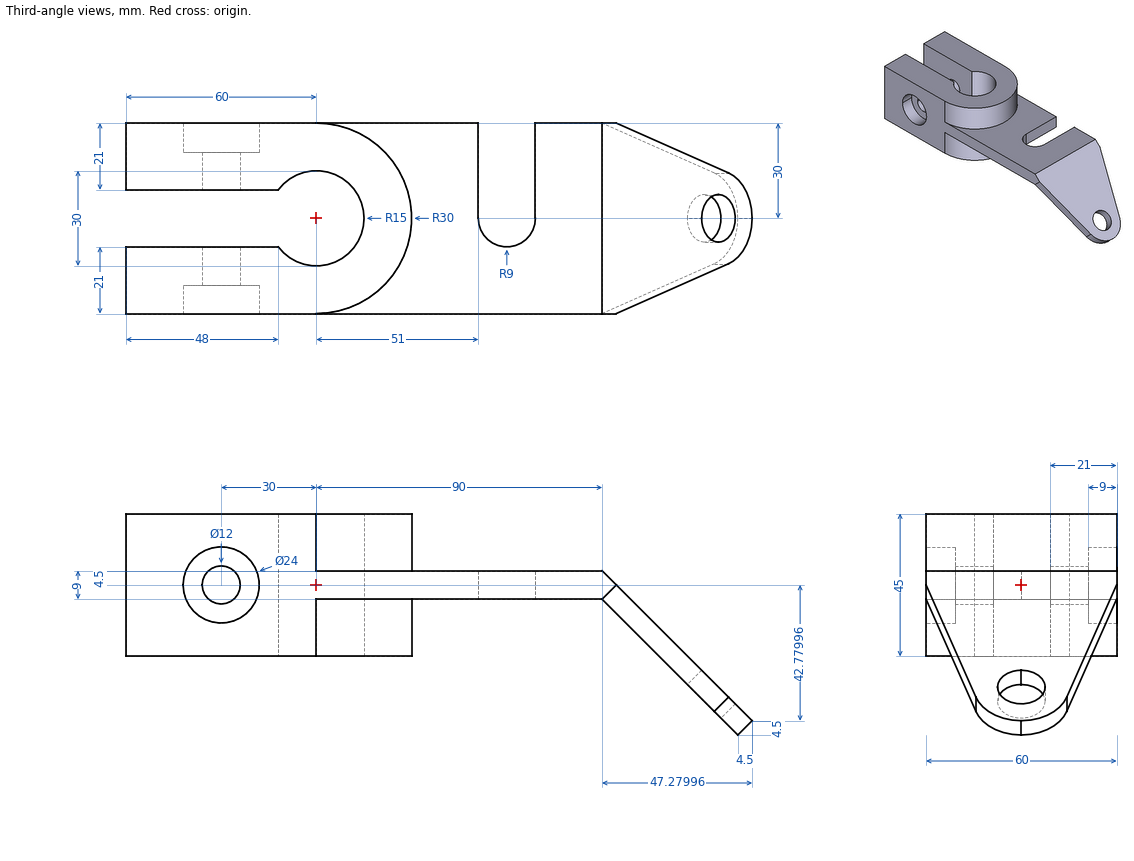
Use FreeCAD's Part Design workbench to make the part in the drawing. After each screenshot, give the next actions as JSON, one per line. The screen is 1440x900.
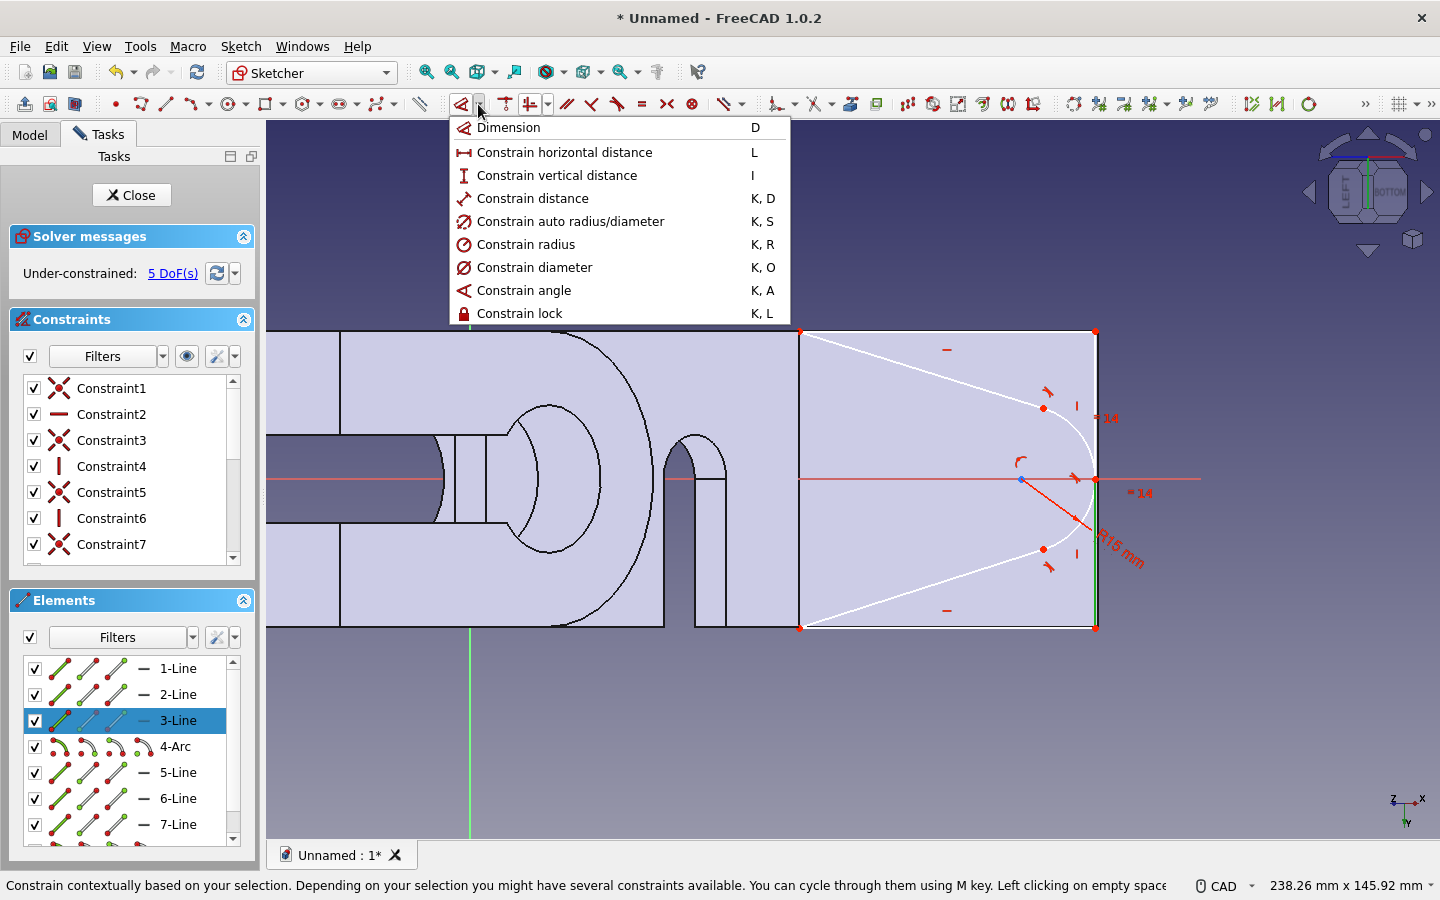
{"action": "left_click", "coordinate": [620, 176]}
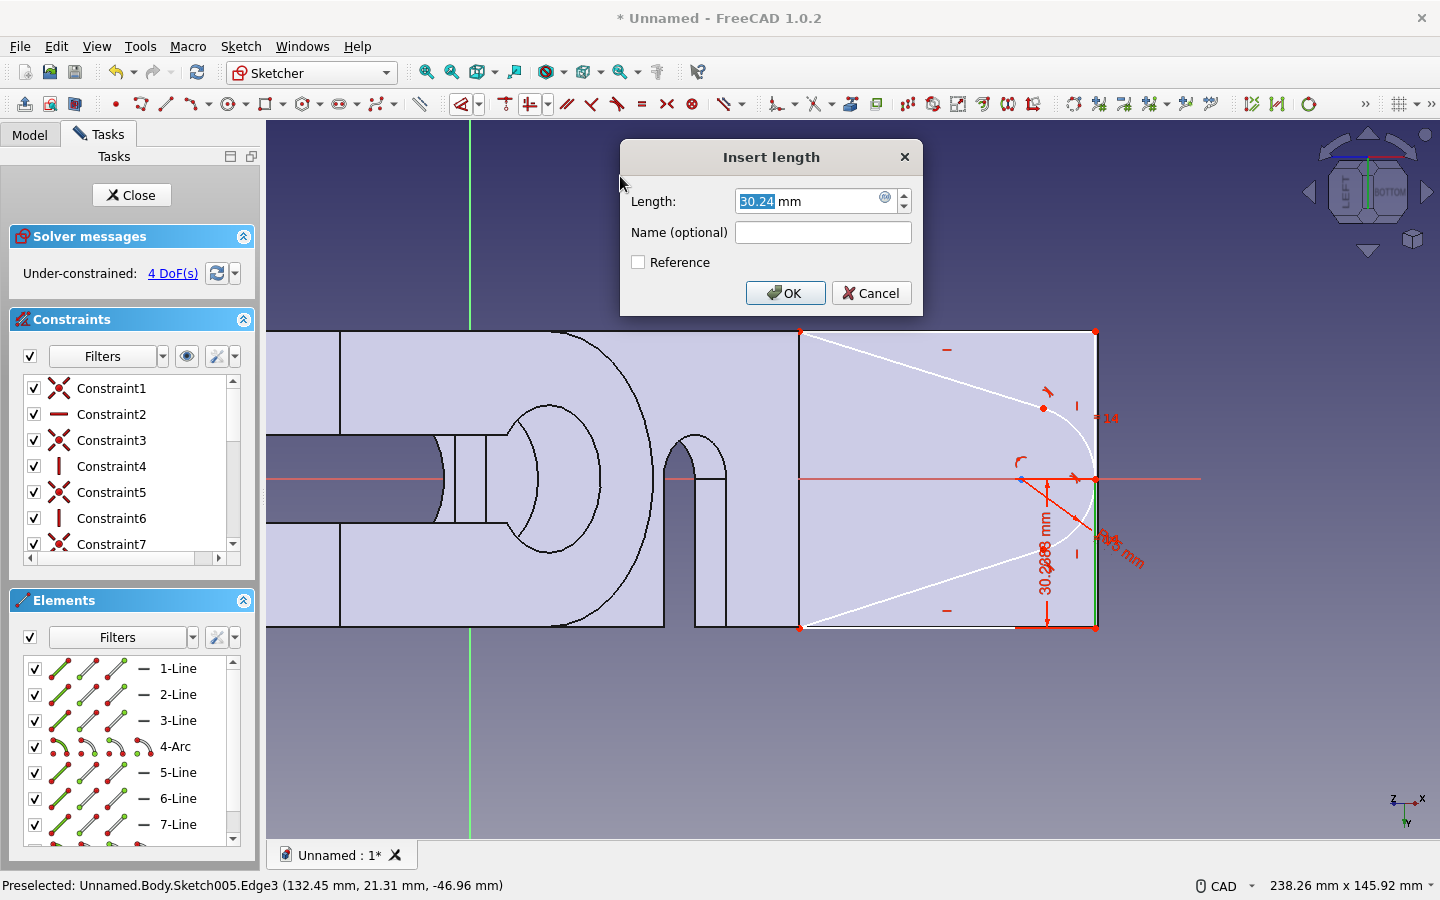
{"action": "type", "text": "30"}
{"action": "key", "text": "Return"}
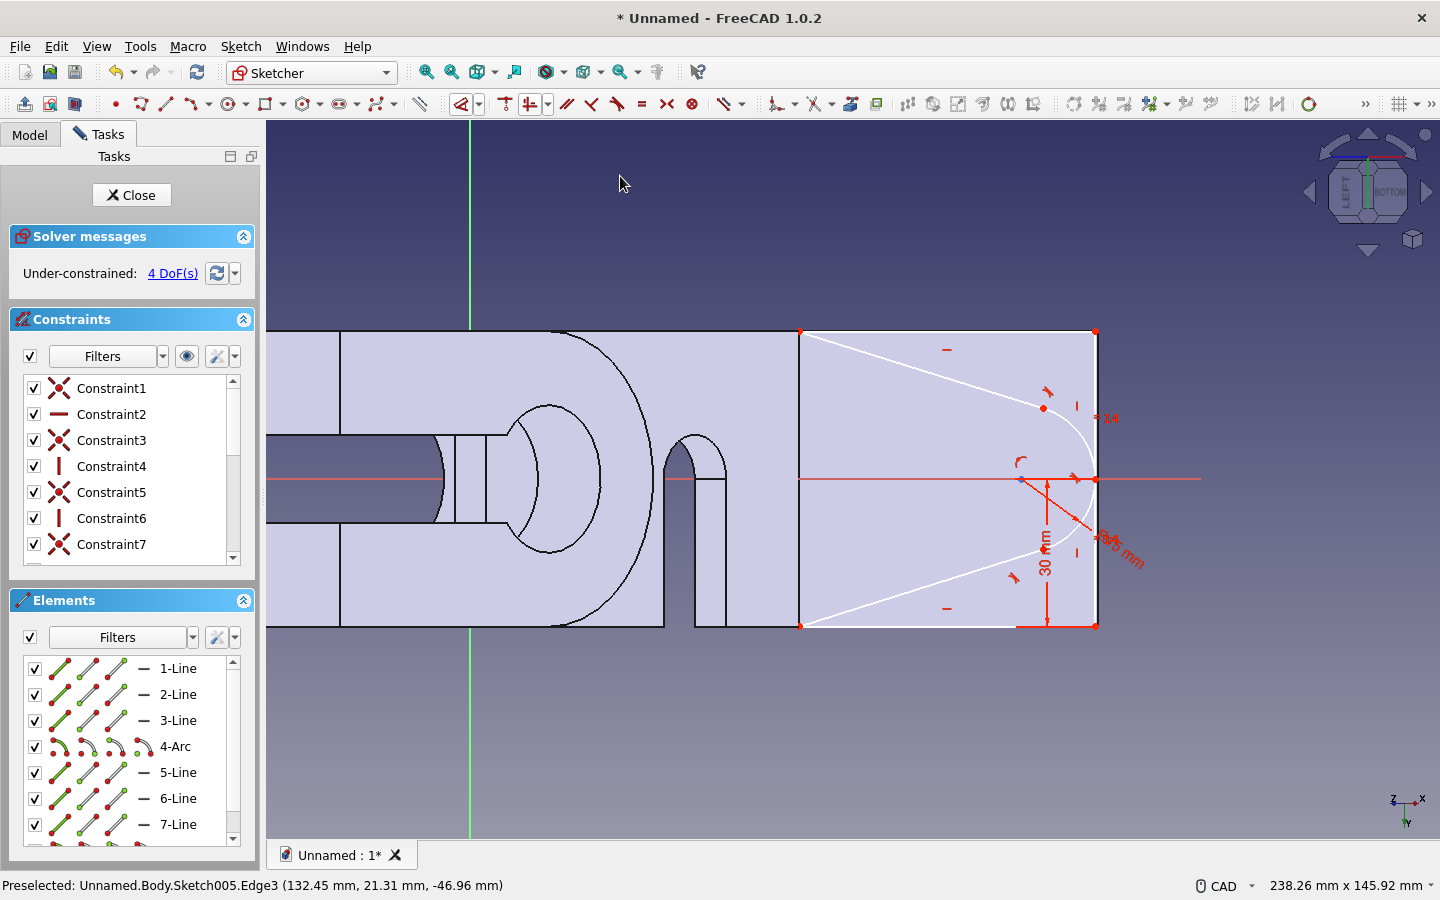
{"action": "left_click", "coordinate": [1095, 435]}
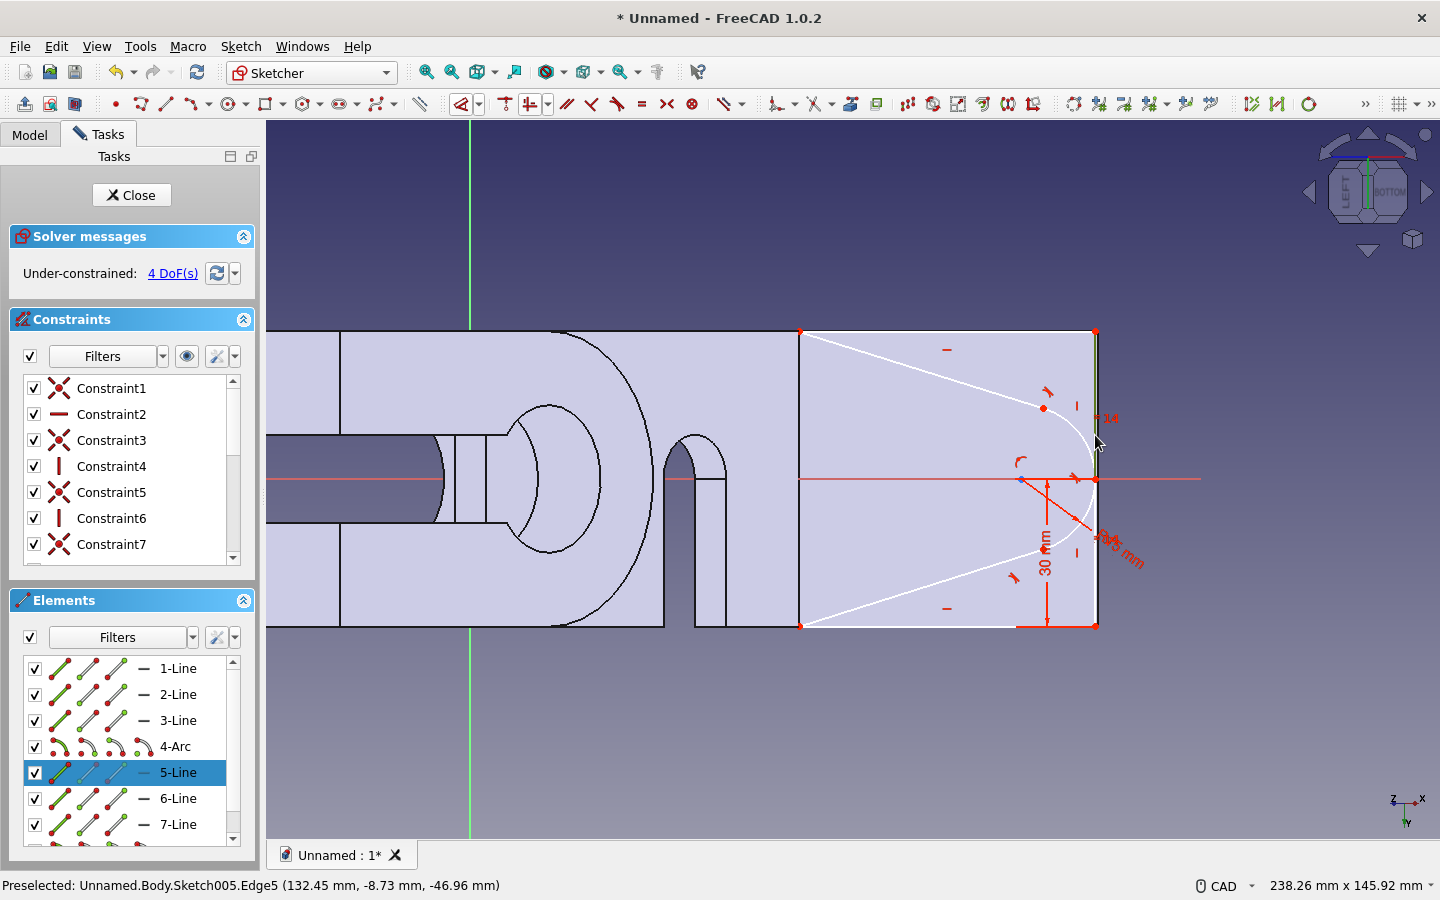
{"action": "left_click", "coordinate": [478, 104]}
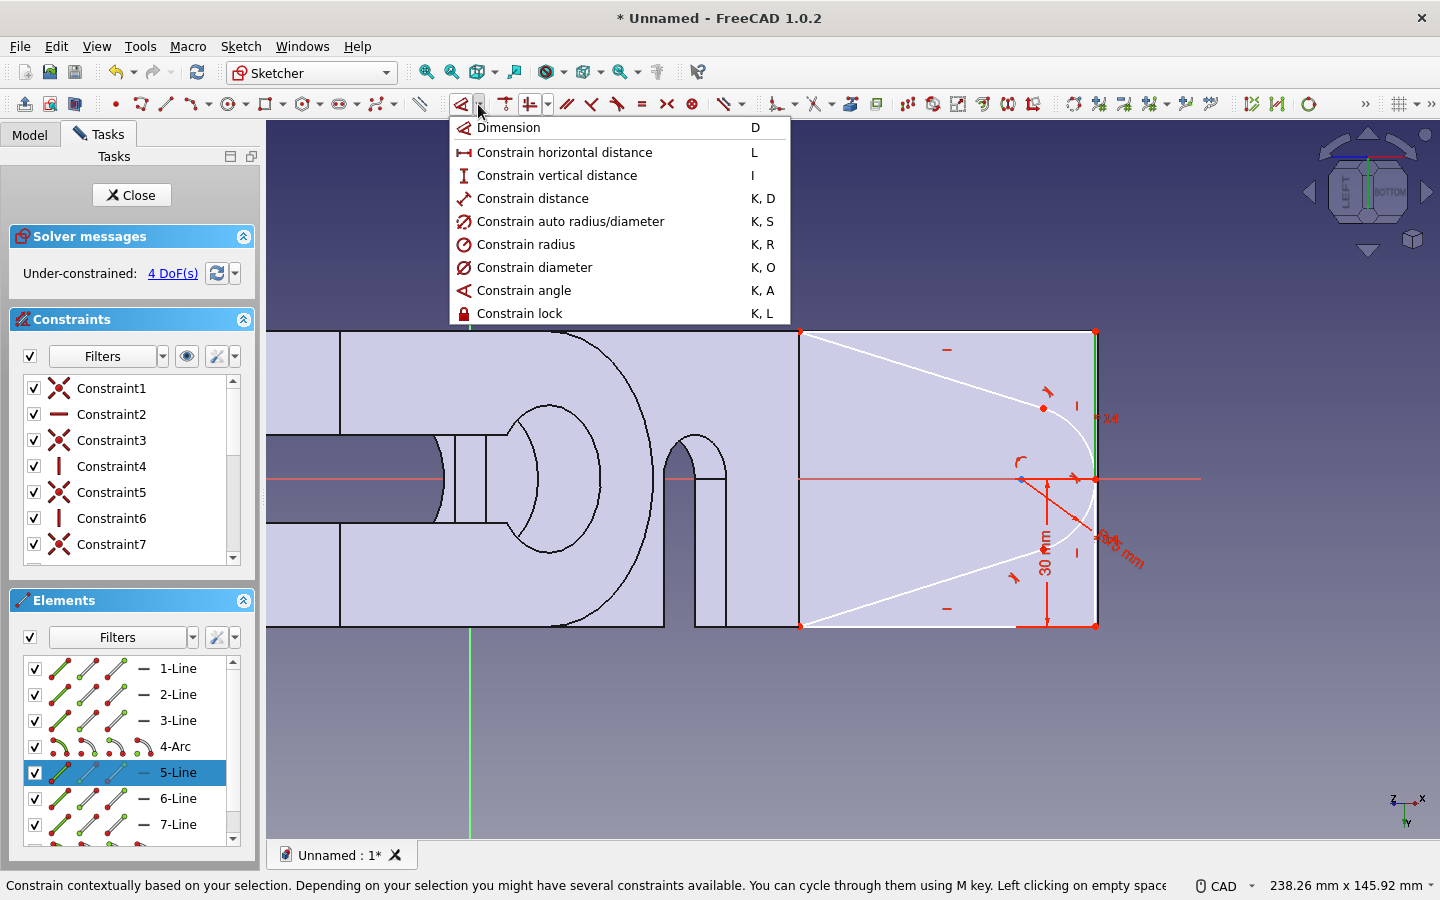
{"action": "left_click", "coordinate": [620, 176]}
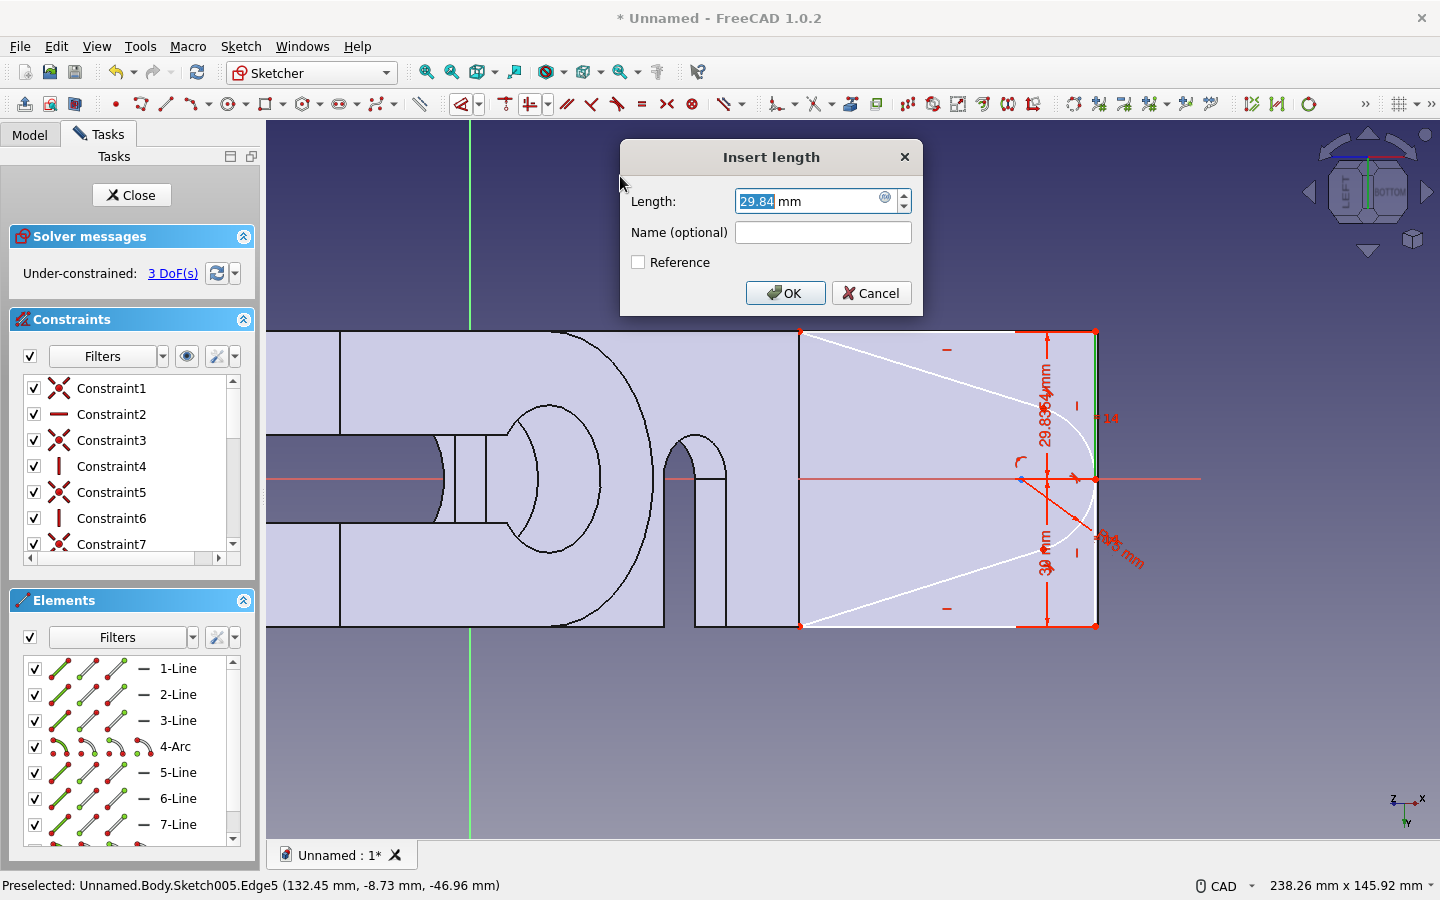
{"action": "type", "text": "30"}
{"action": "key", "text": "Return"}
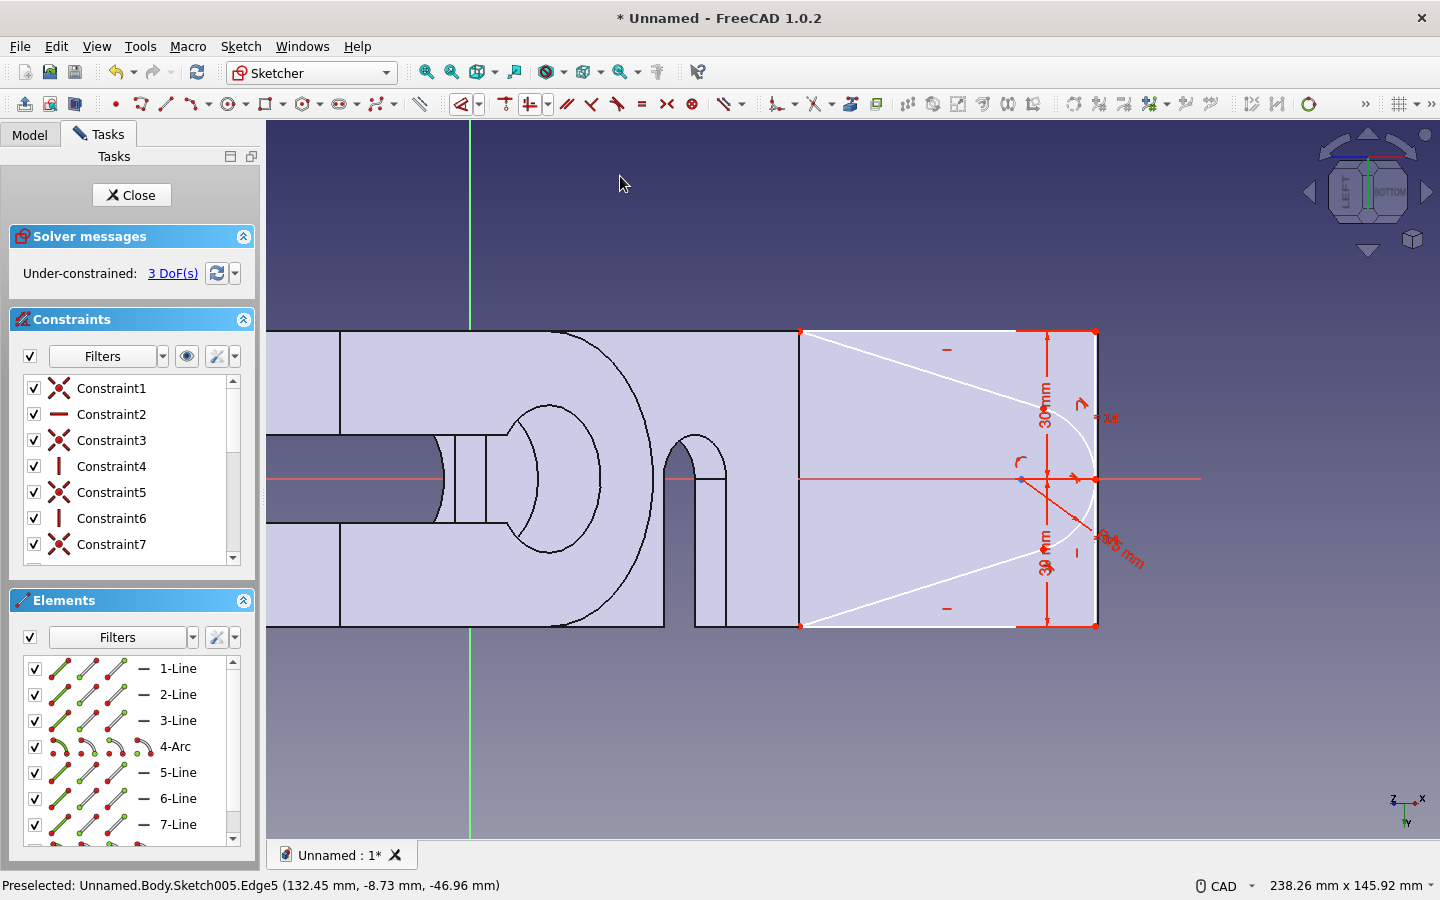
{"action": "left_click", "coordinate": [888, 627]}